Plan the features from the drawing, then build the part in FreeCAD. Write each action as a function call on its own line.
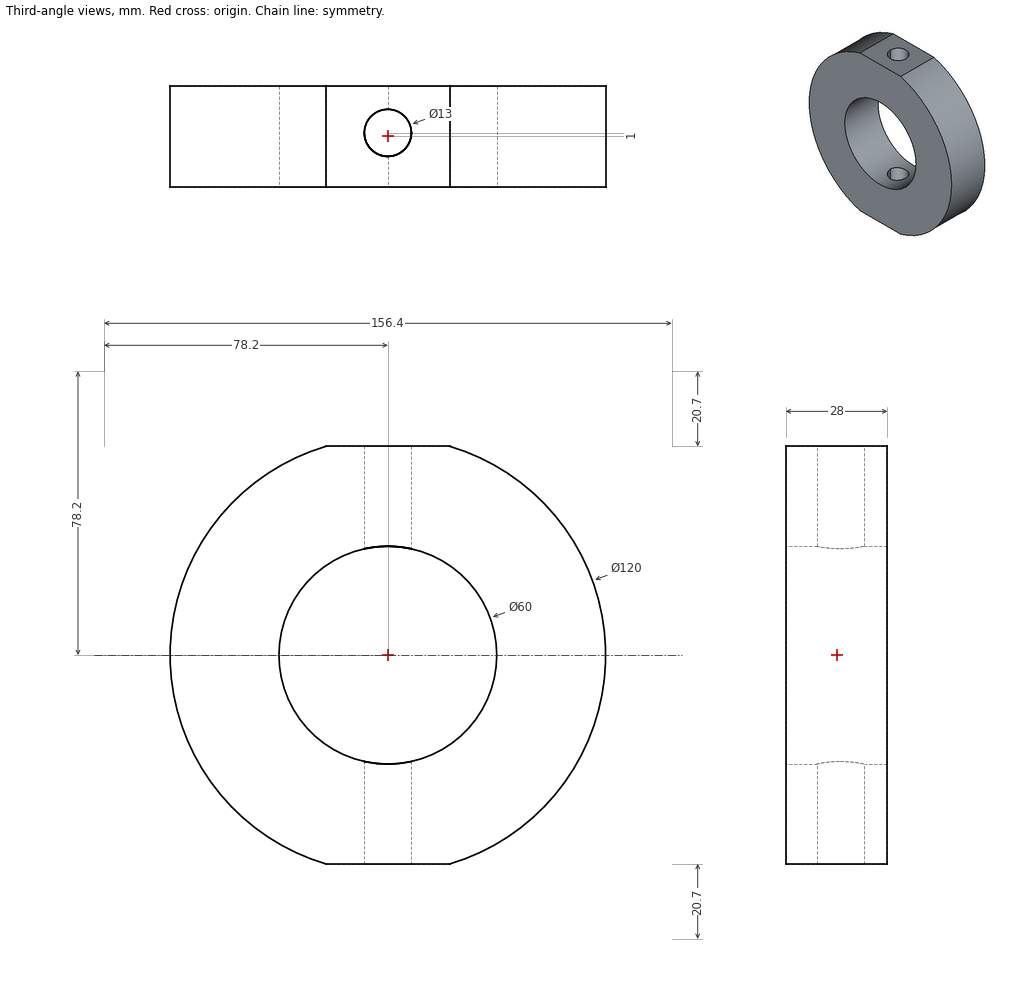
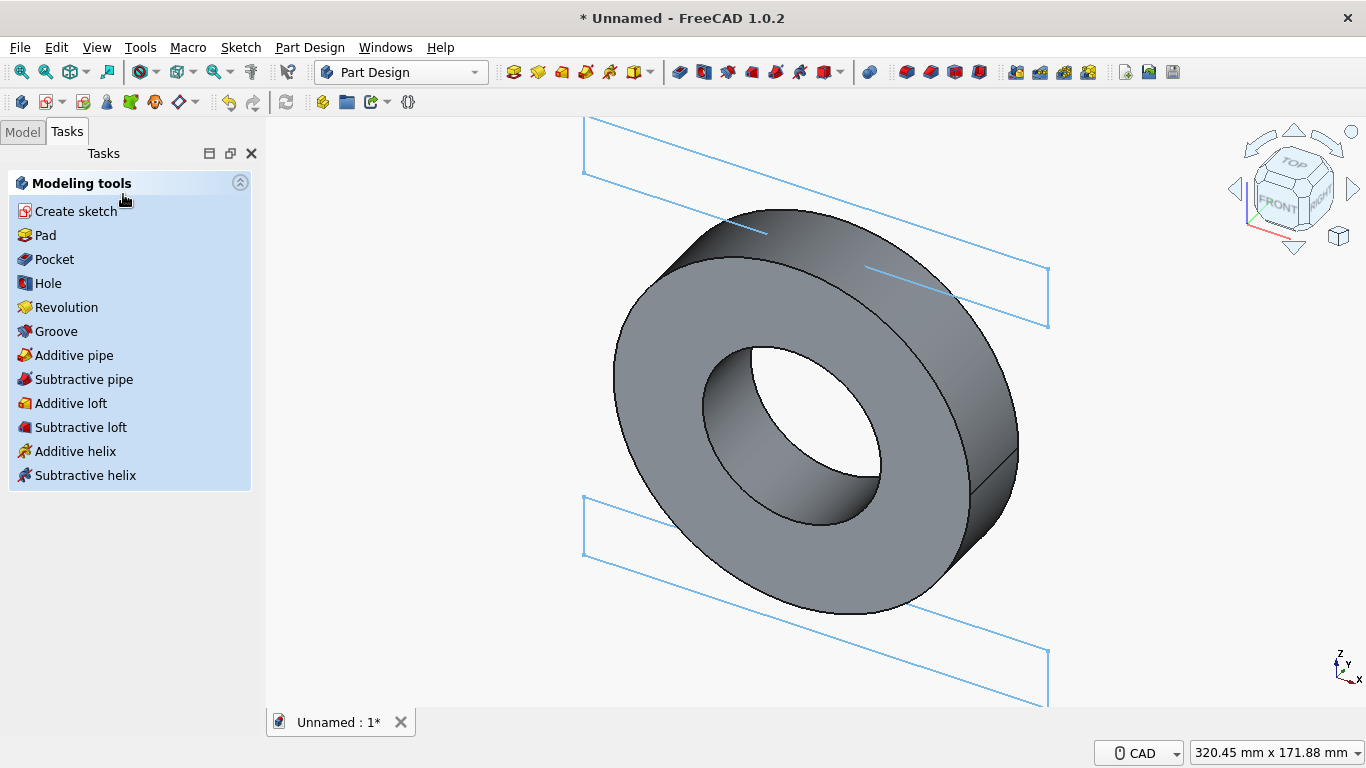
click(680, 72)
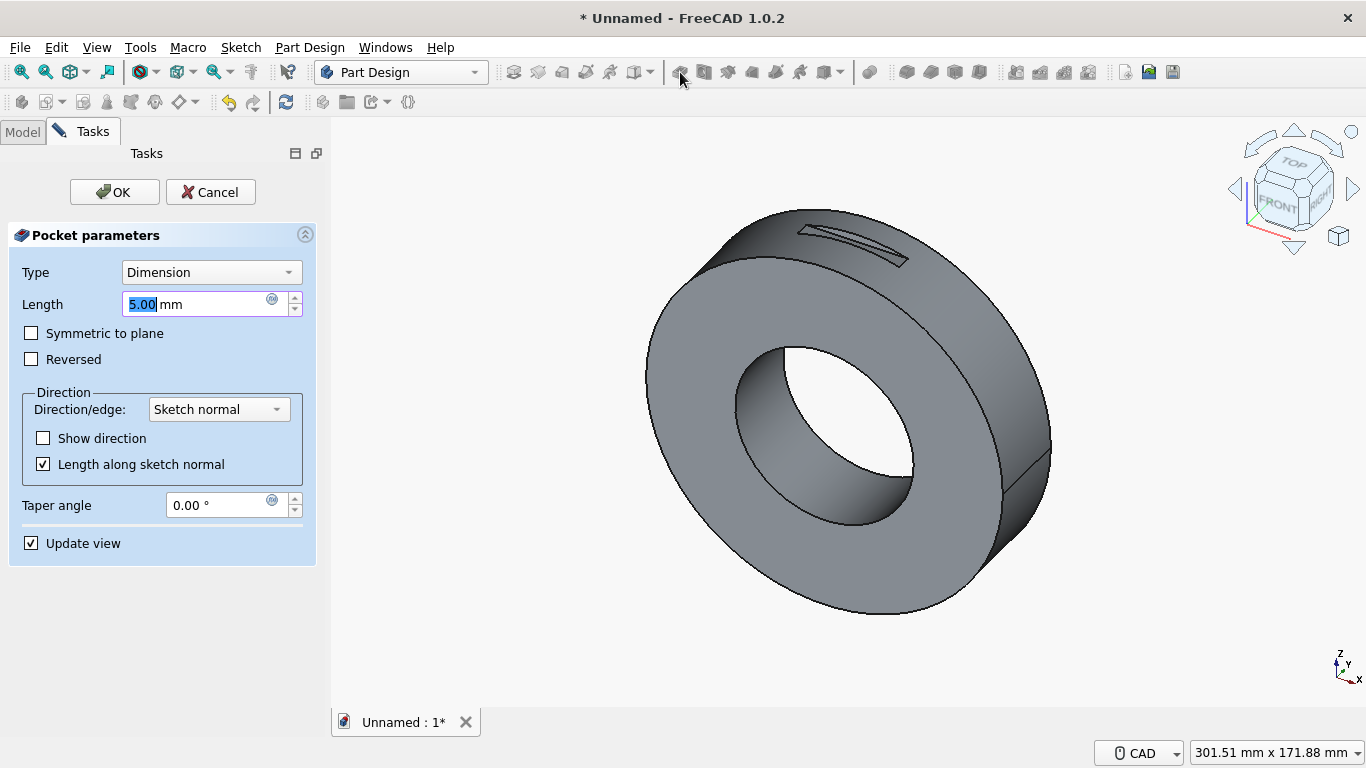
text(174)
key(Tab)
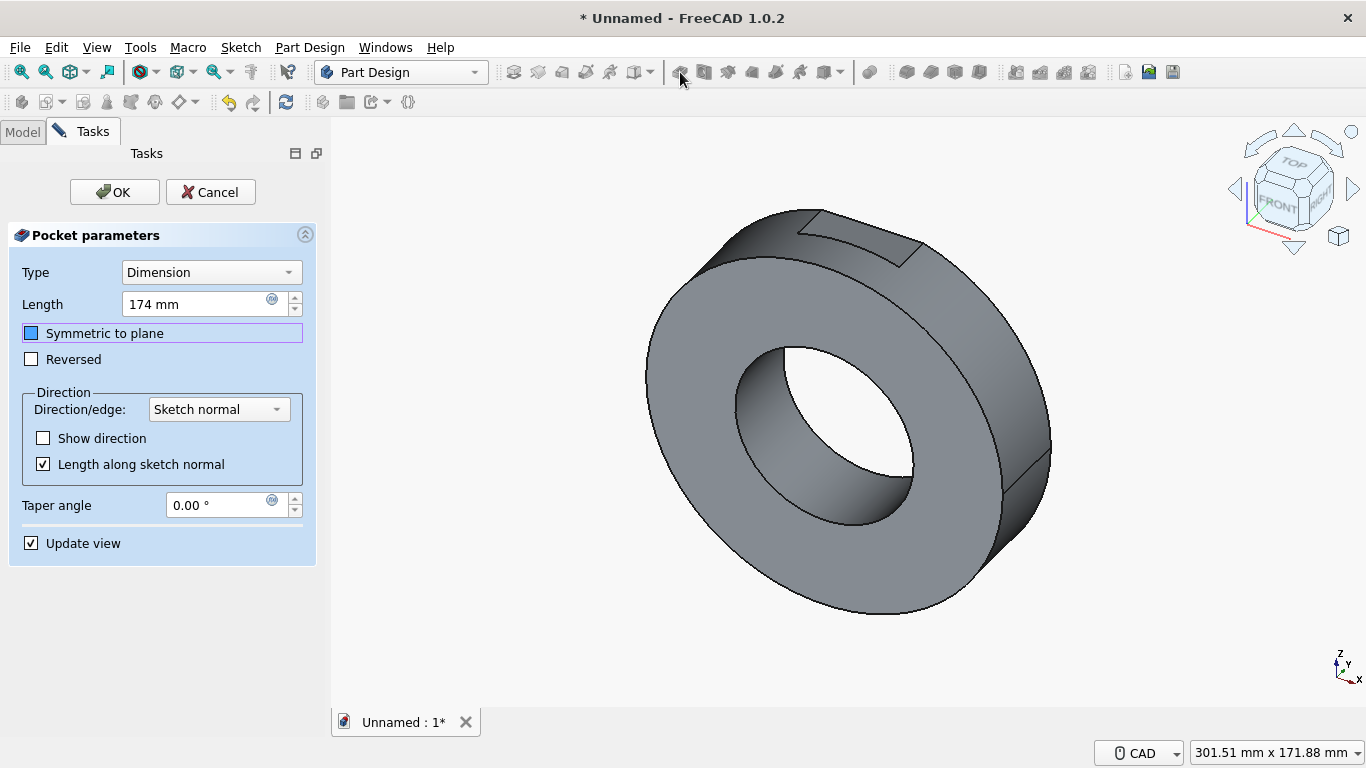
click(30, 333)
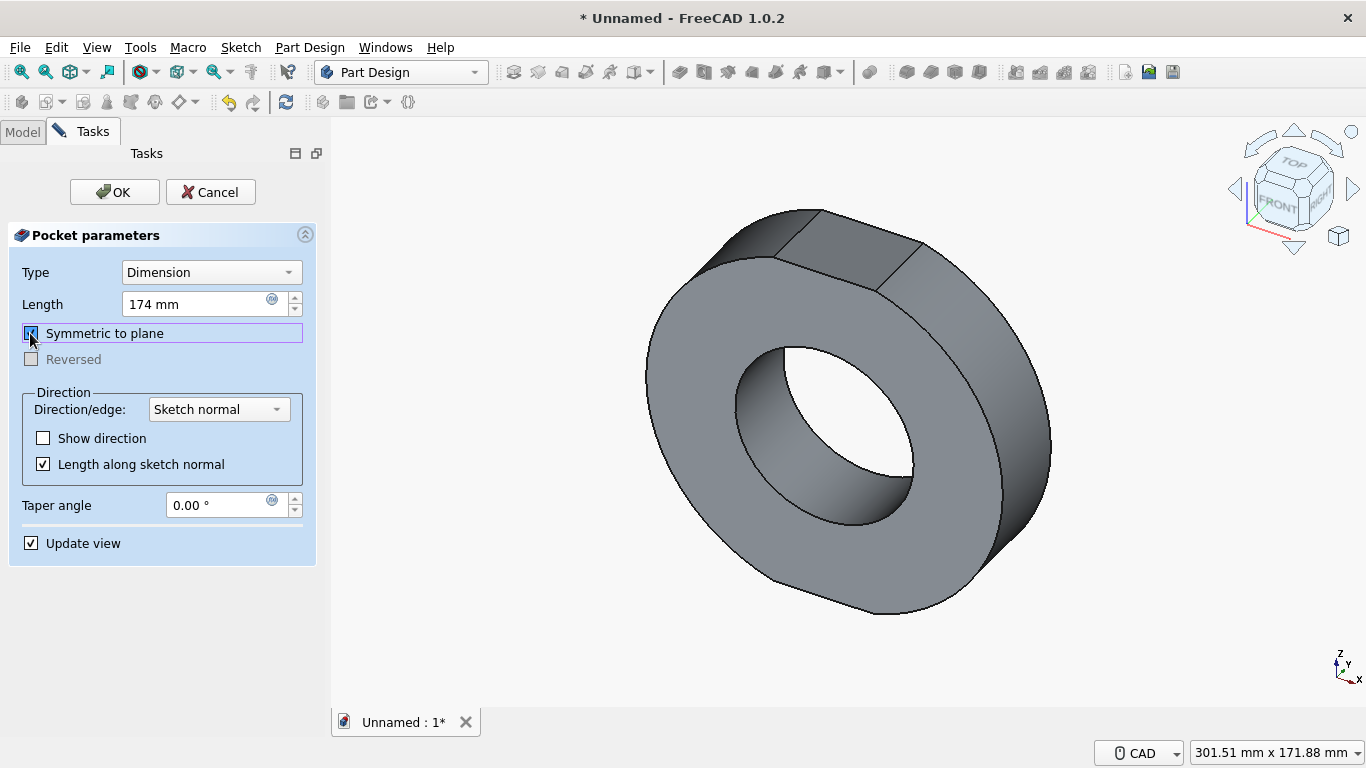
click(115, 192)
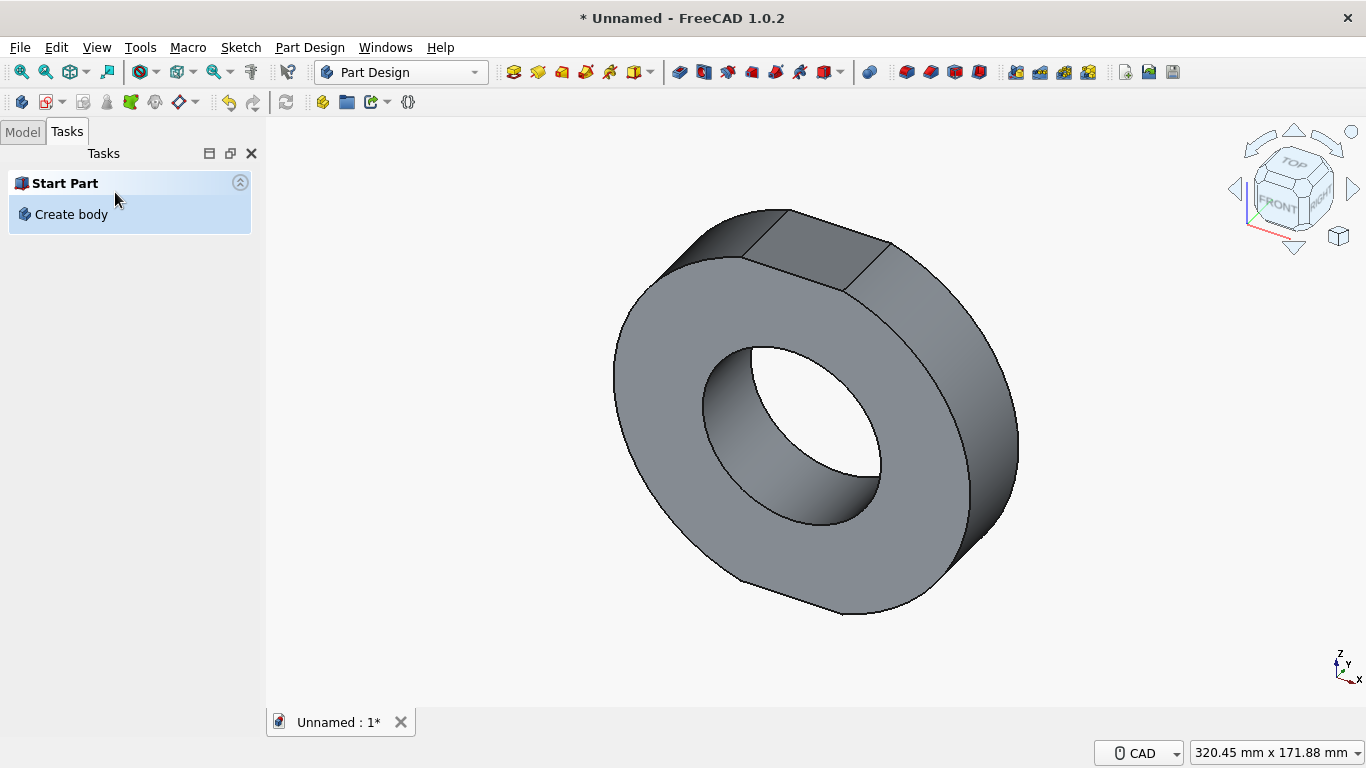
click(816, 249)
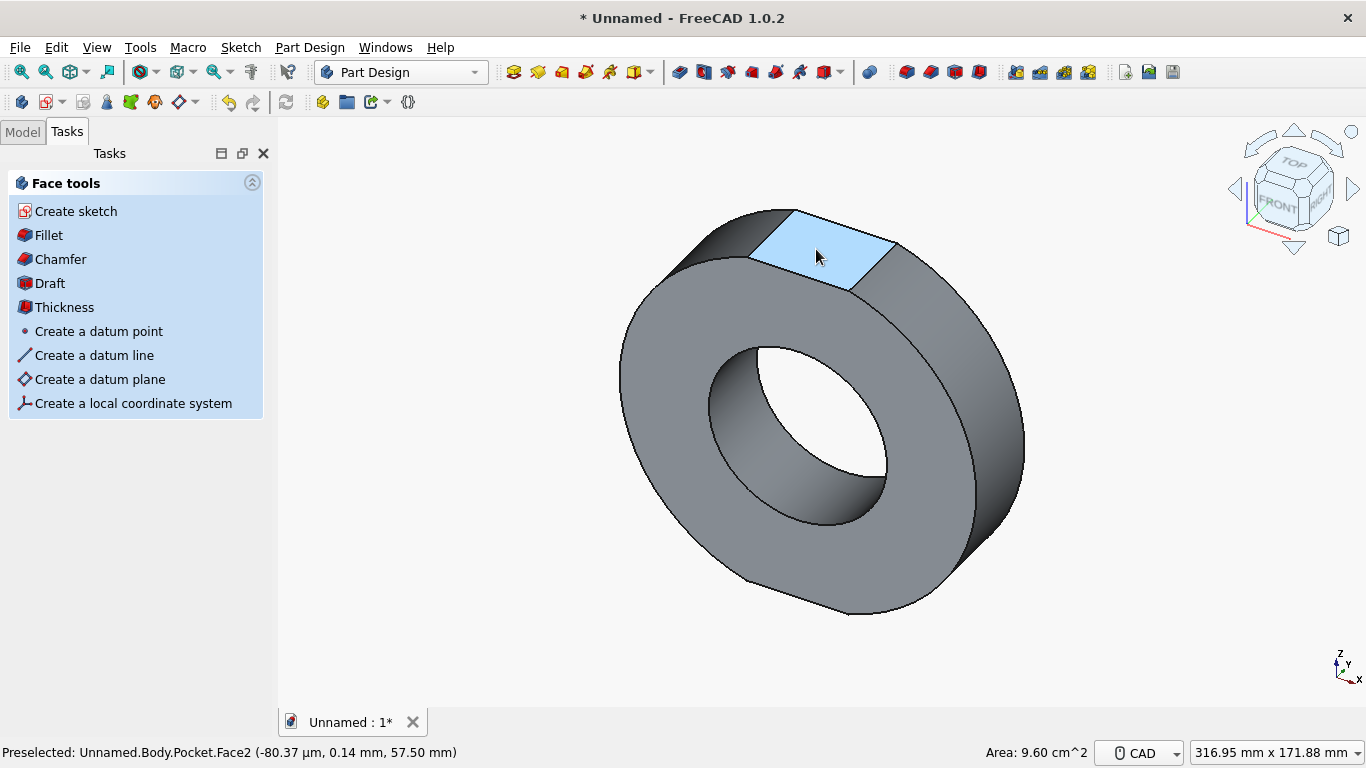
click(46, 102)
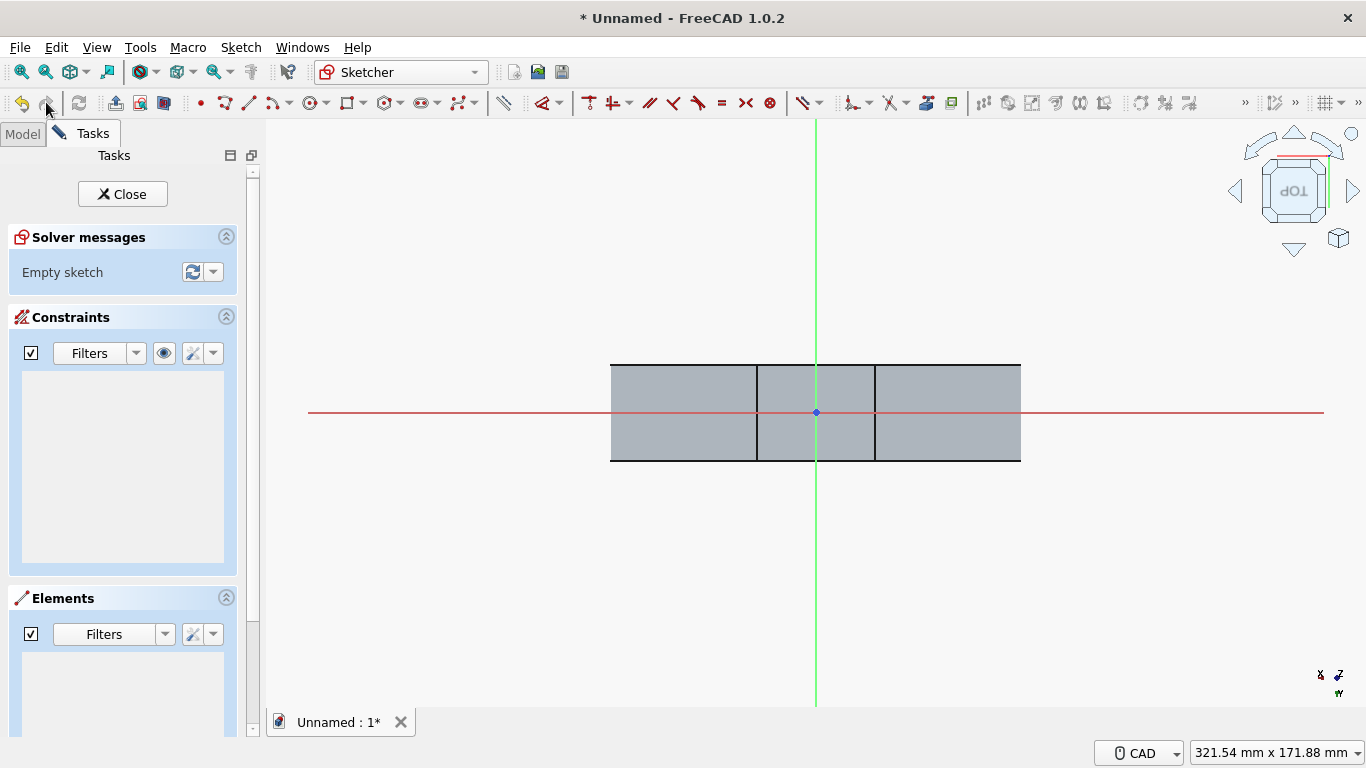
scroll(825, 417, up, 11)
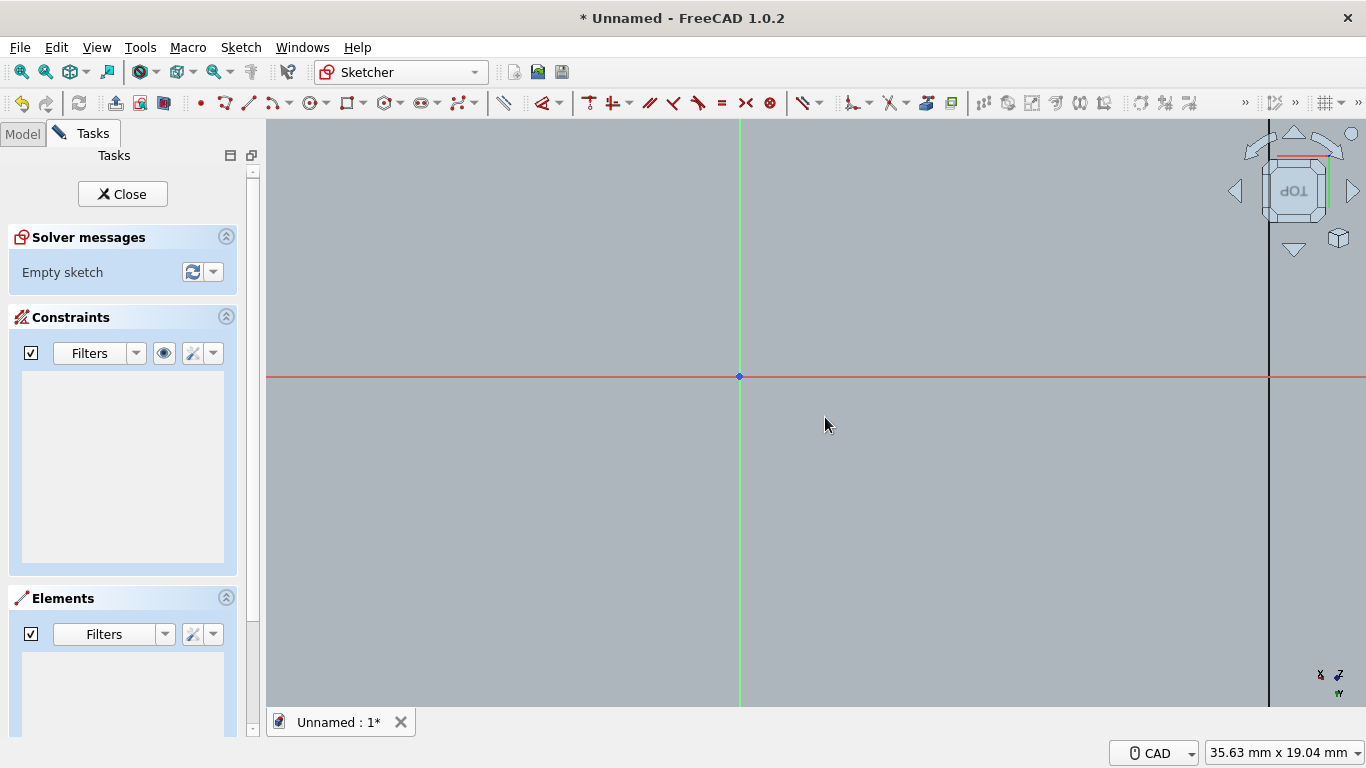
key(g)
key(c)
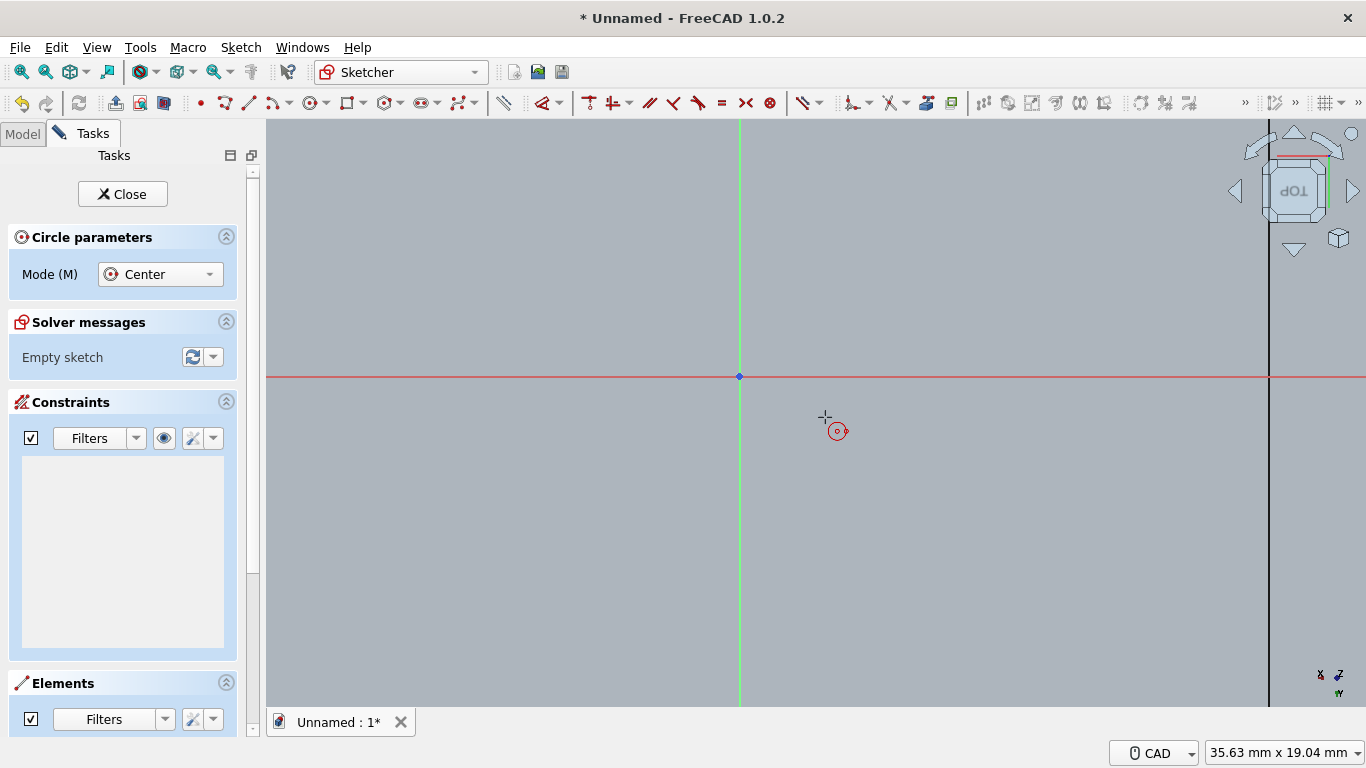
click(740, 408)
move(882, 266)